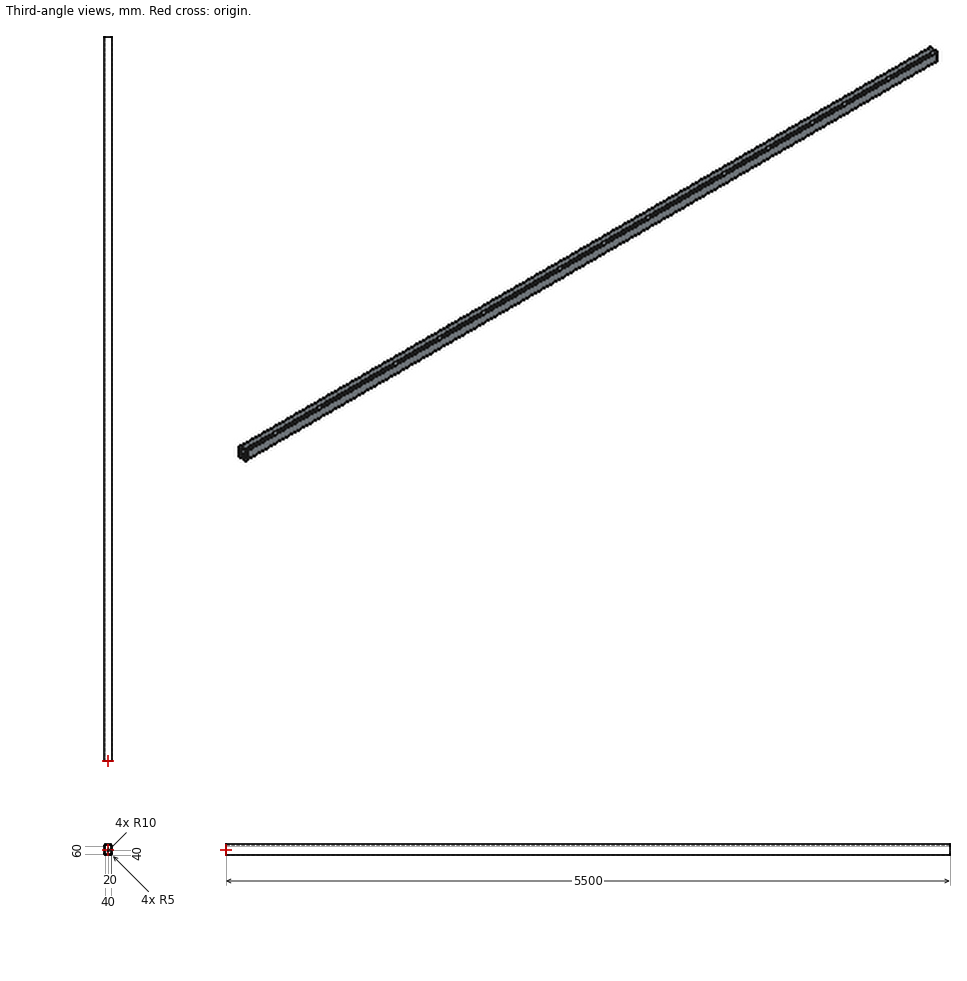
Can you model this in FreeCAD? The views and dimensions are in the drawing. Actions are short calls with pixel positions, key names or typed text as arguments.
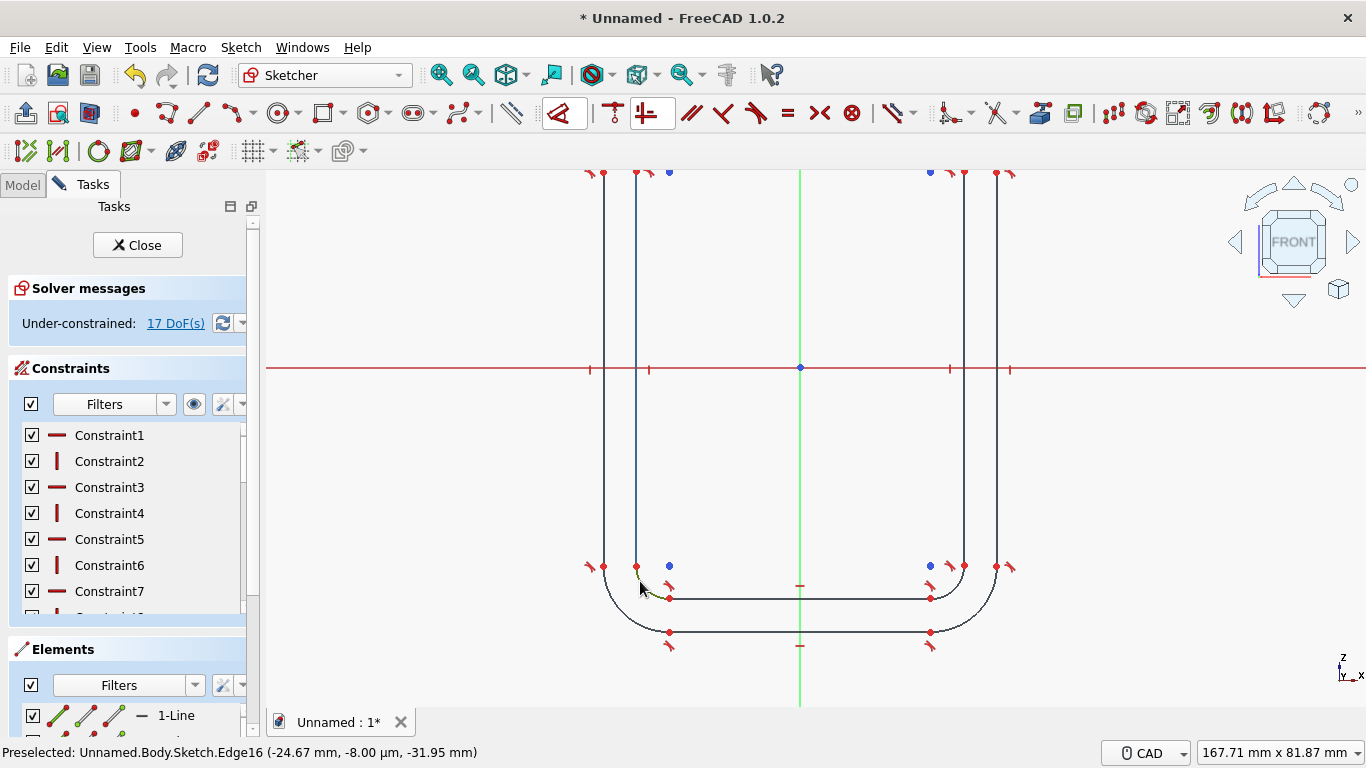
click(756, 114)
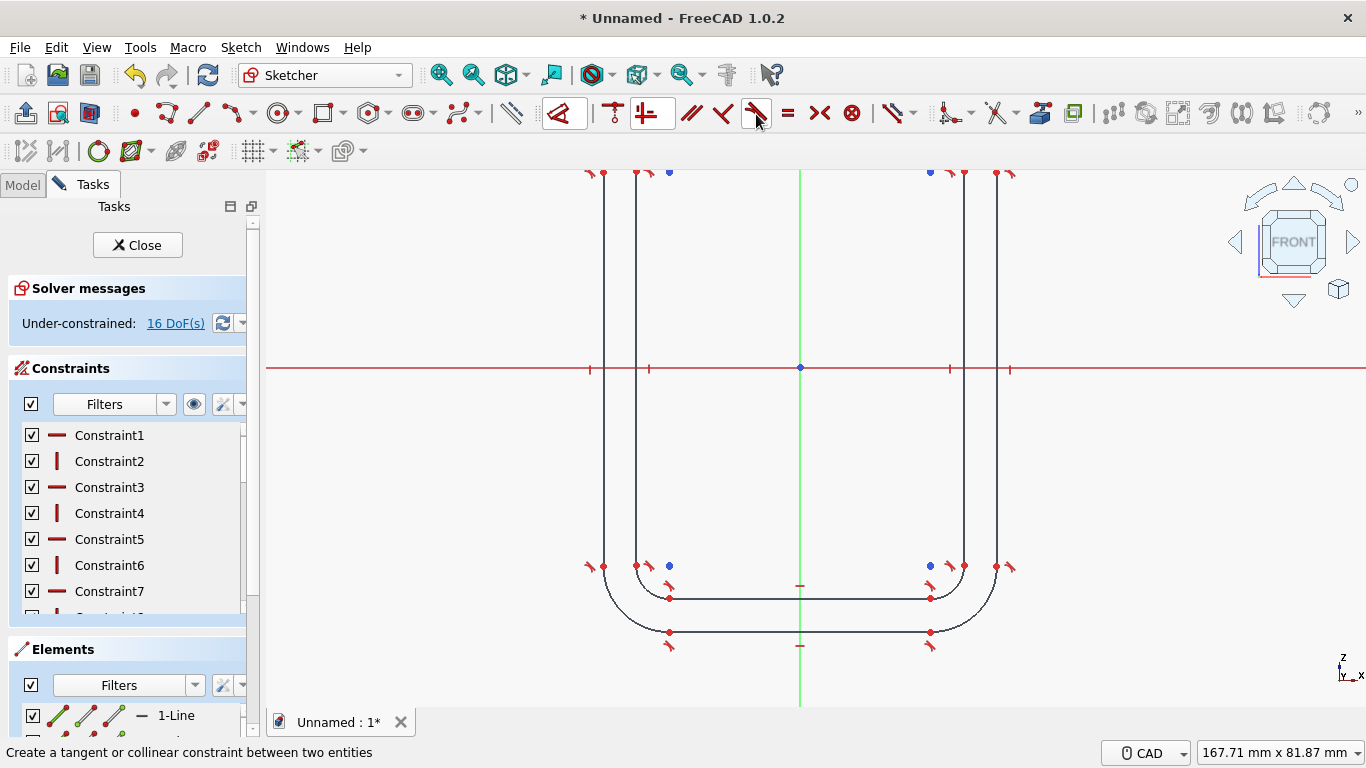
click(961, 625)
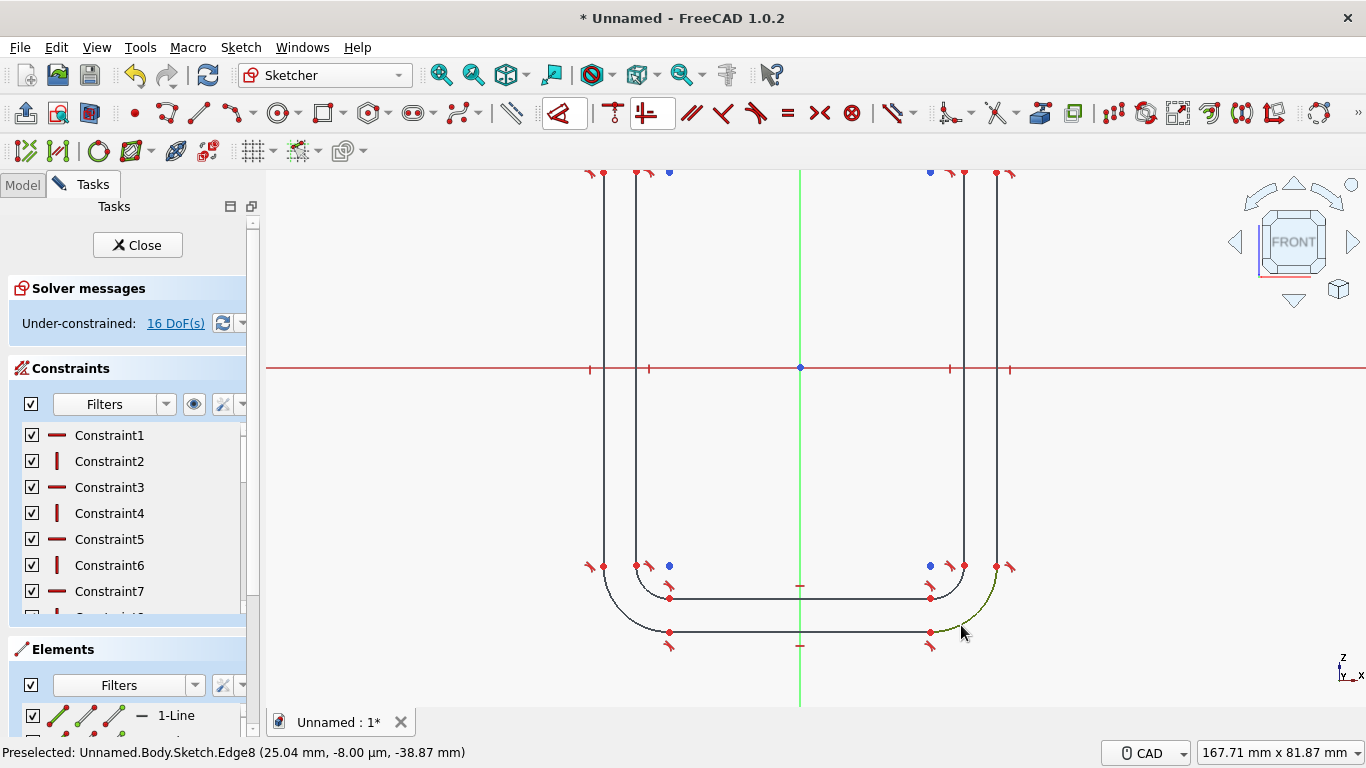
click(946, 595)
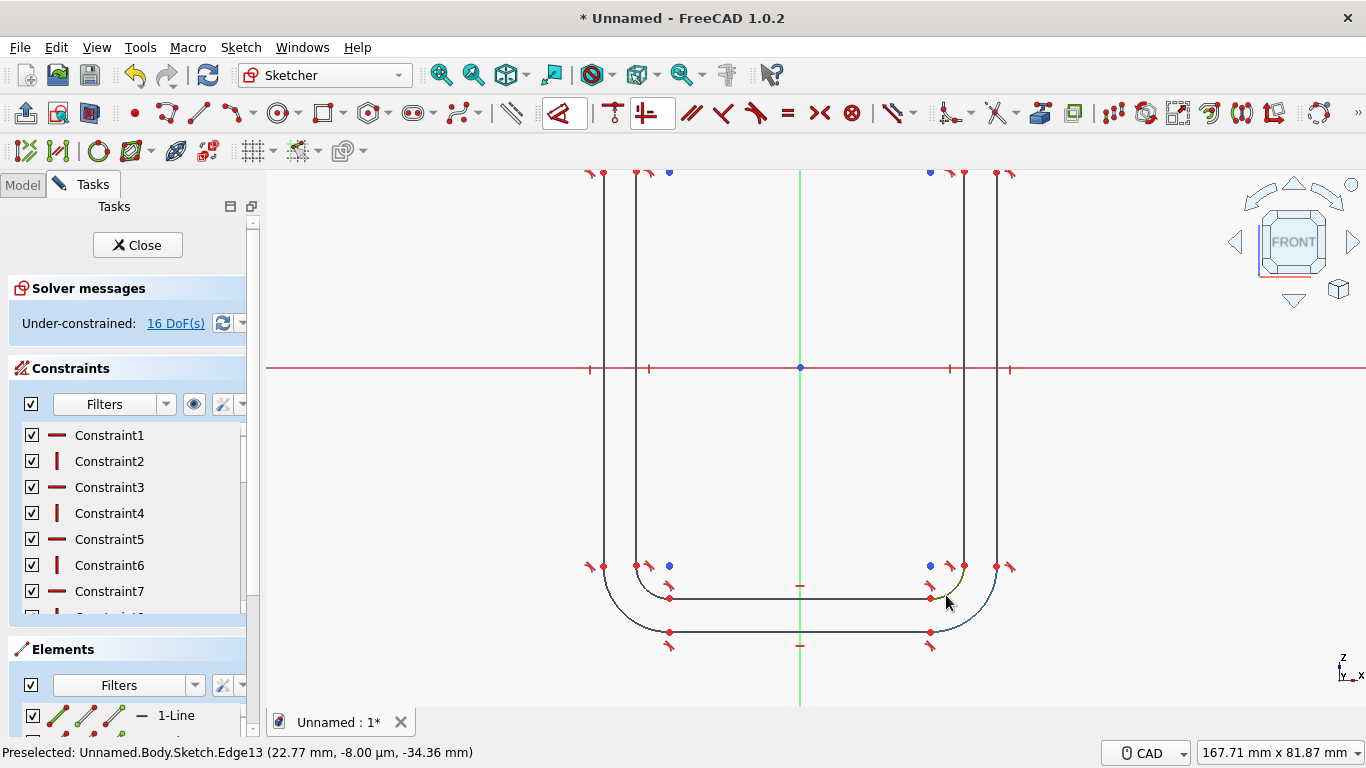
click(614, 114)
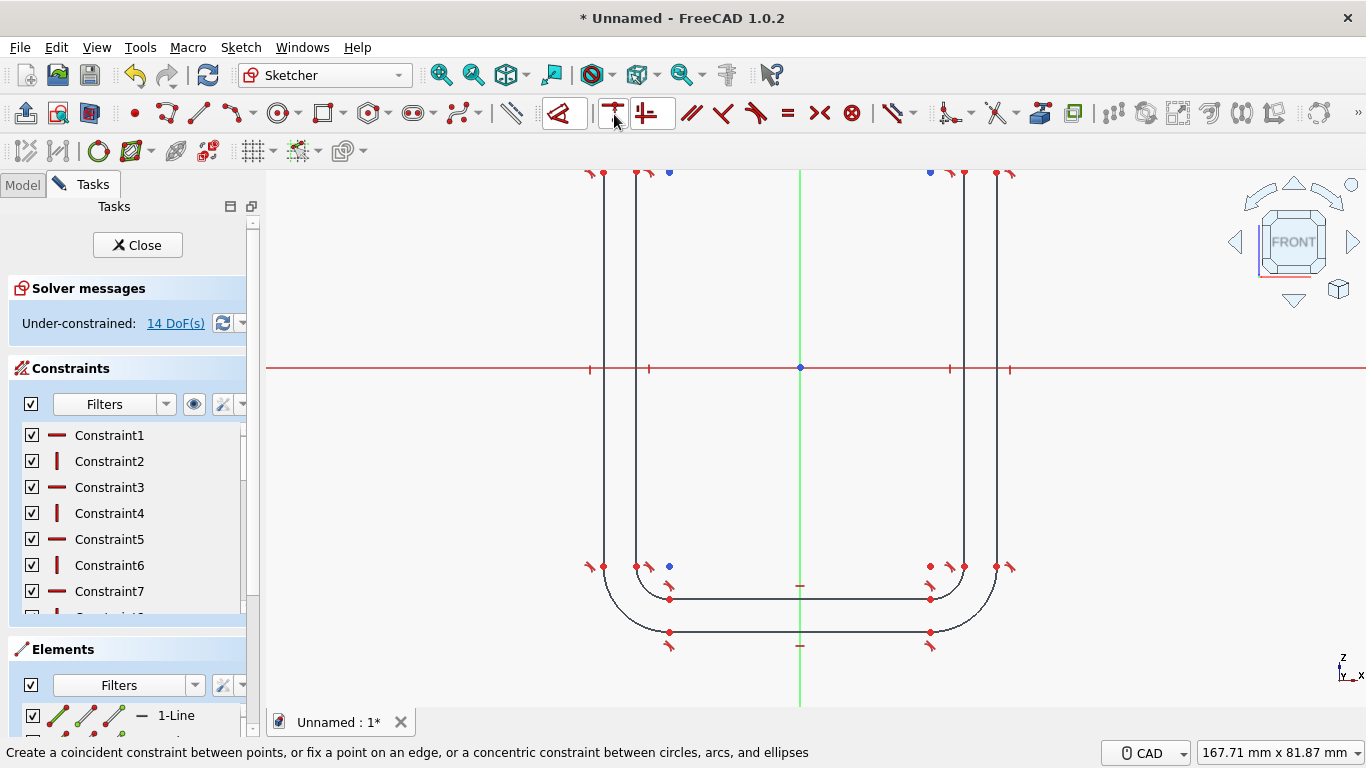
scroll(640, 582, down, 2)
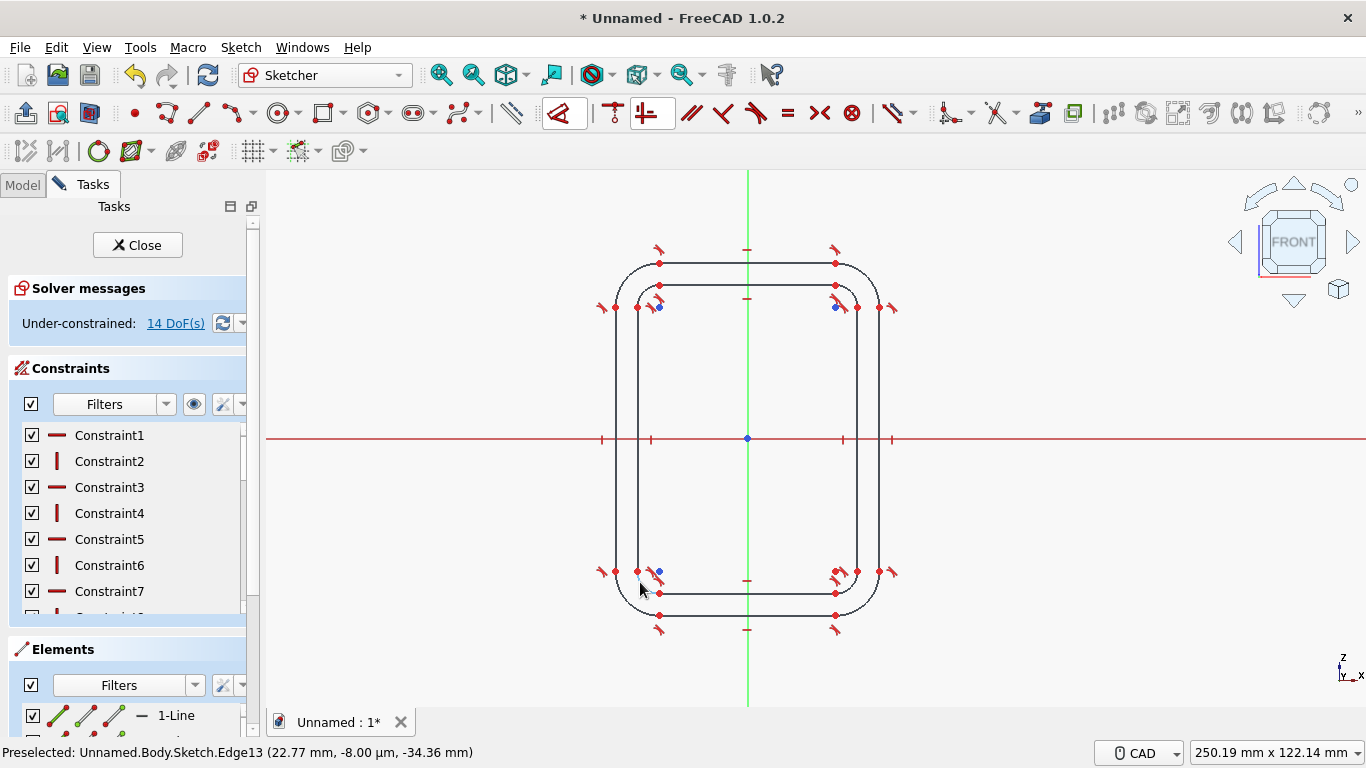
click(875, 287)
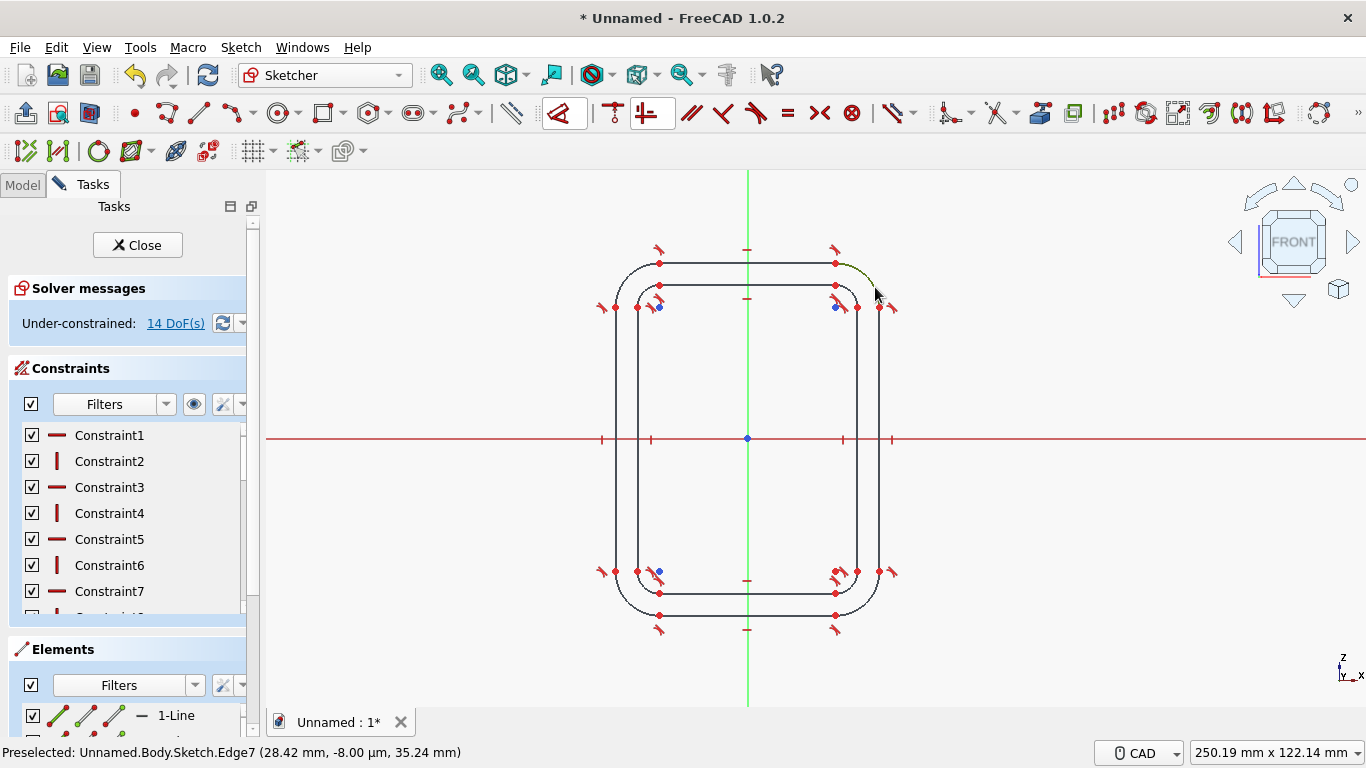
scroll(855, 297, up, 2)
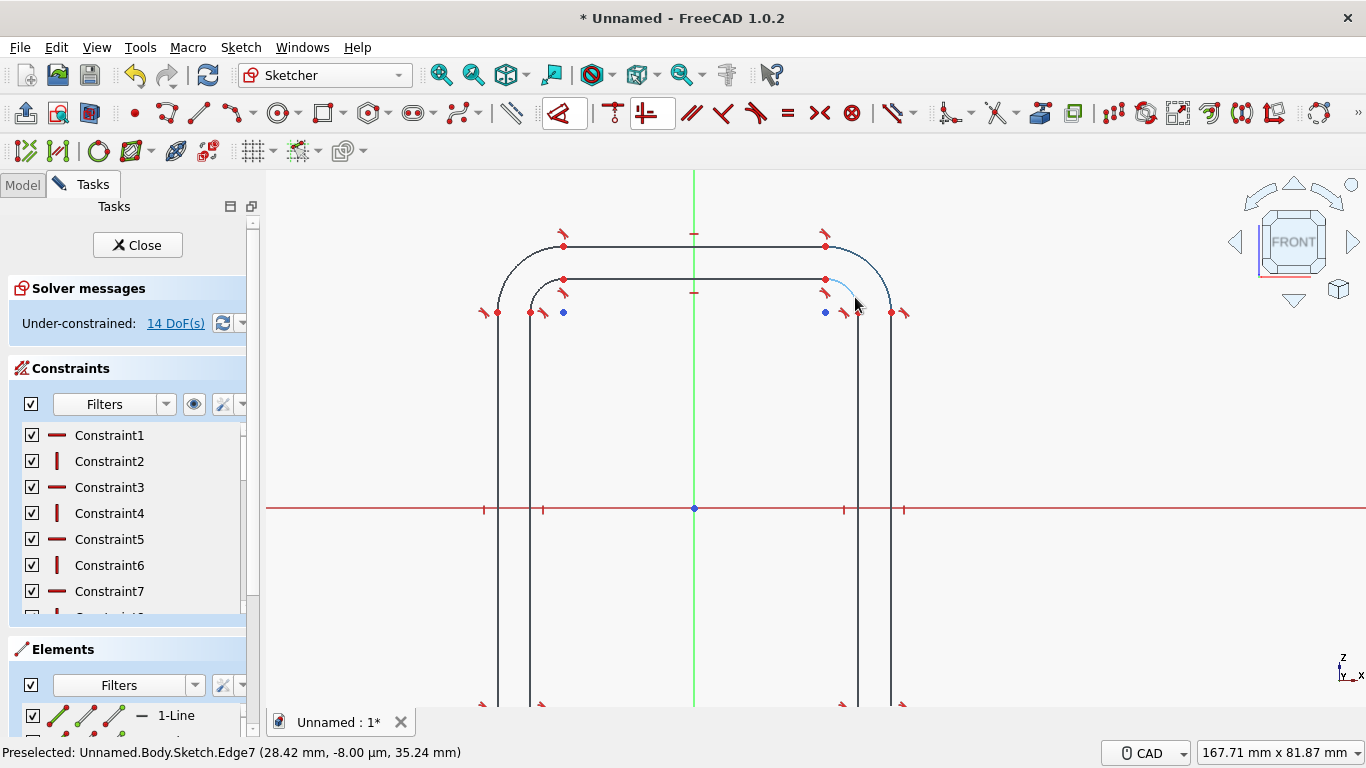
click(855, 297)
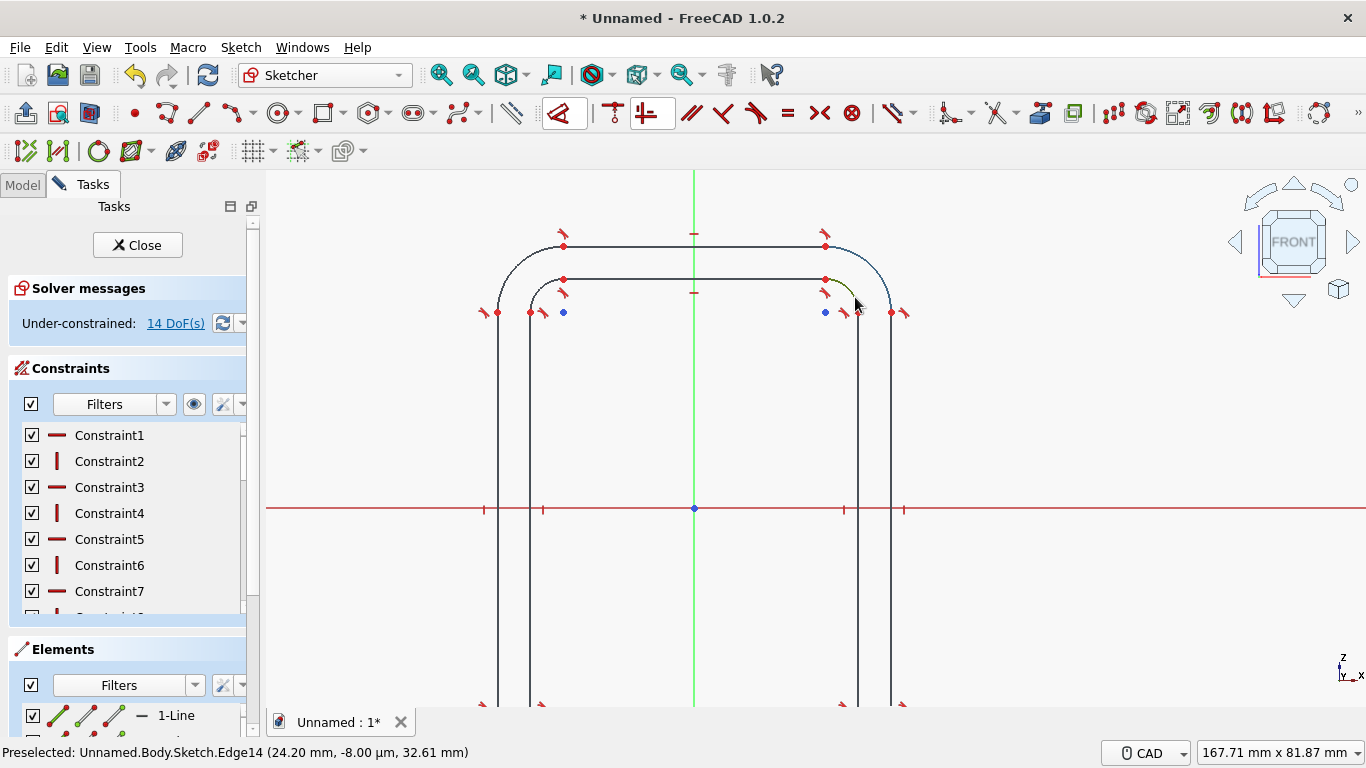
click(614, 114)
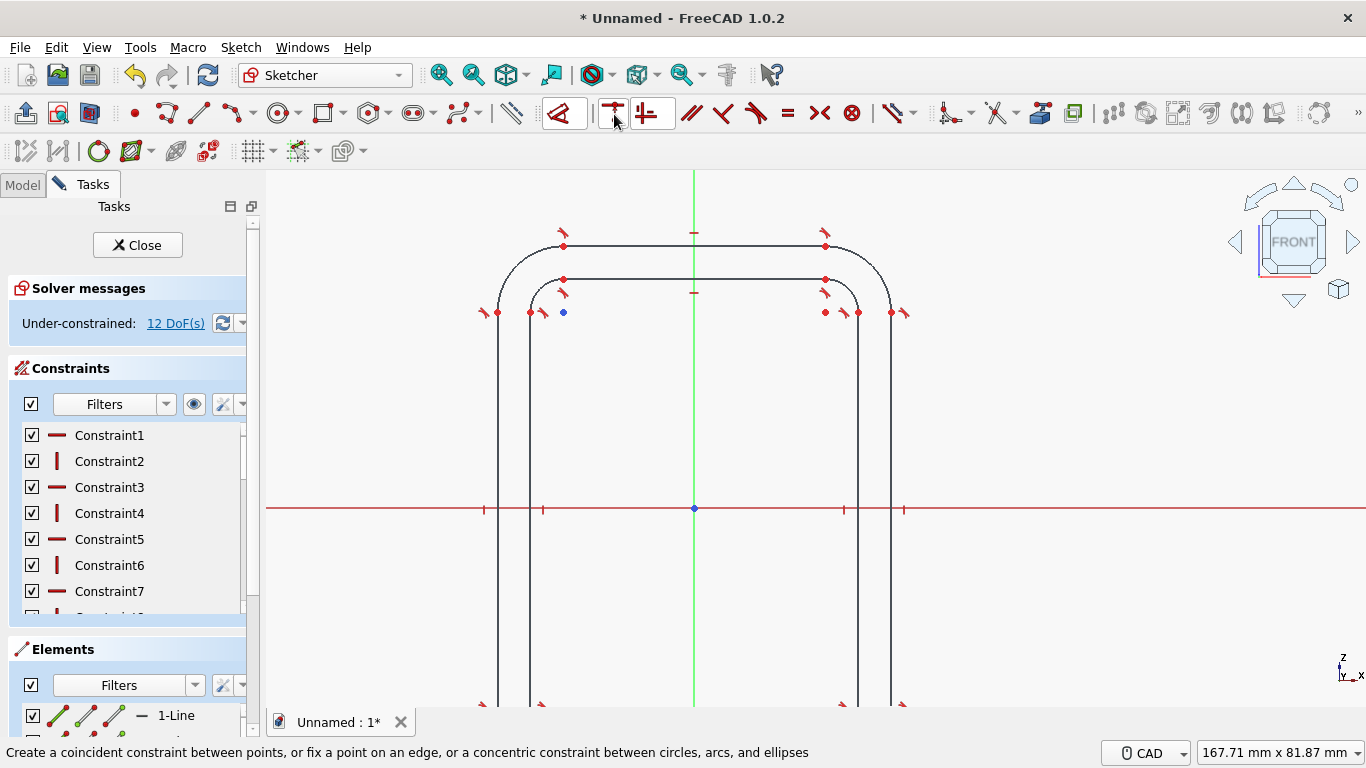
click(534, 254)